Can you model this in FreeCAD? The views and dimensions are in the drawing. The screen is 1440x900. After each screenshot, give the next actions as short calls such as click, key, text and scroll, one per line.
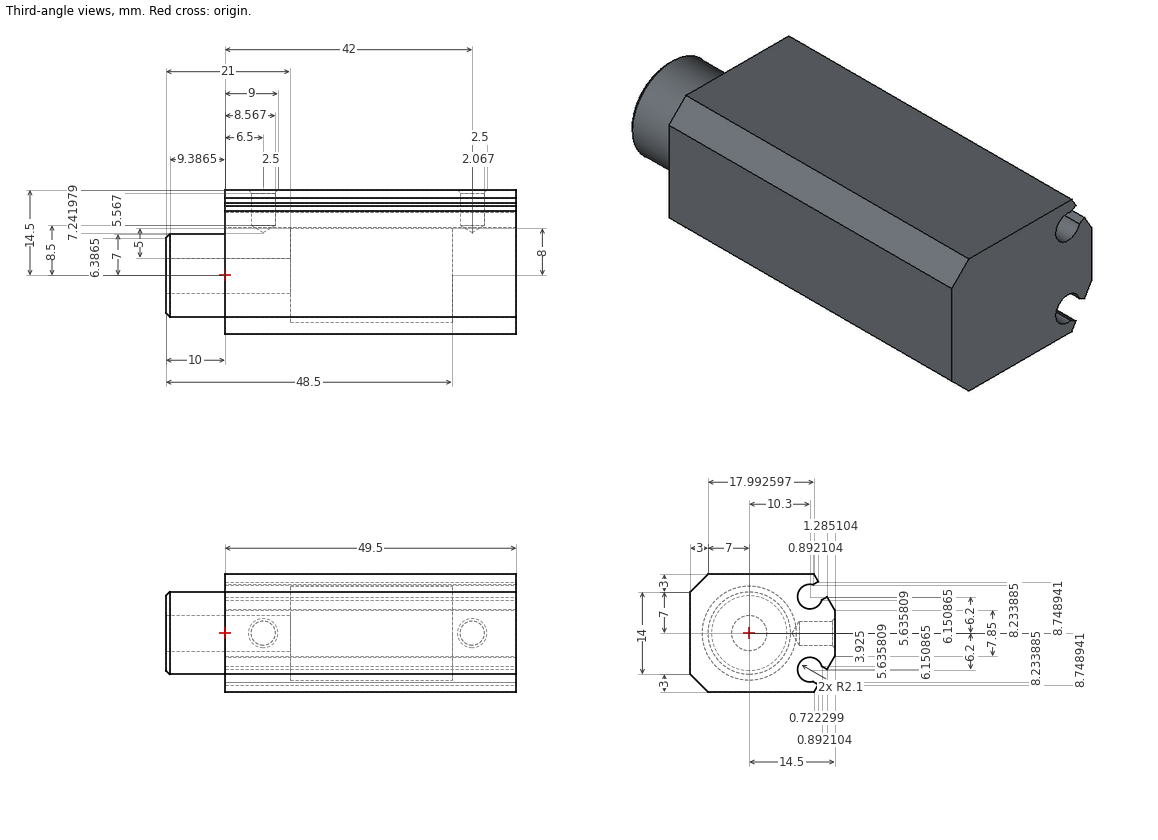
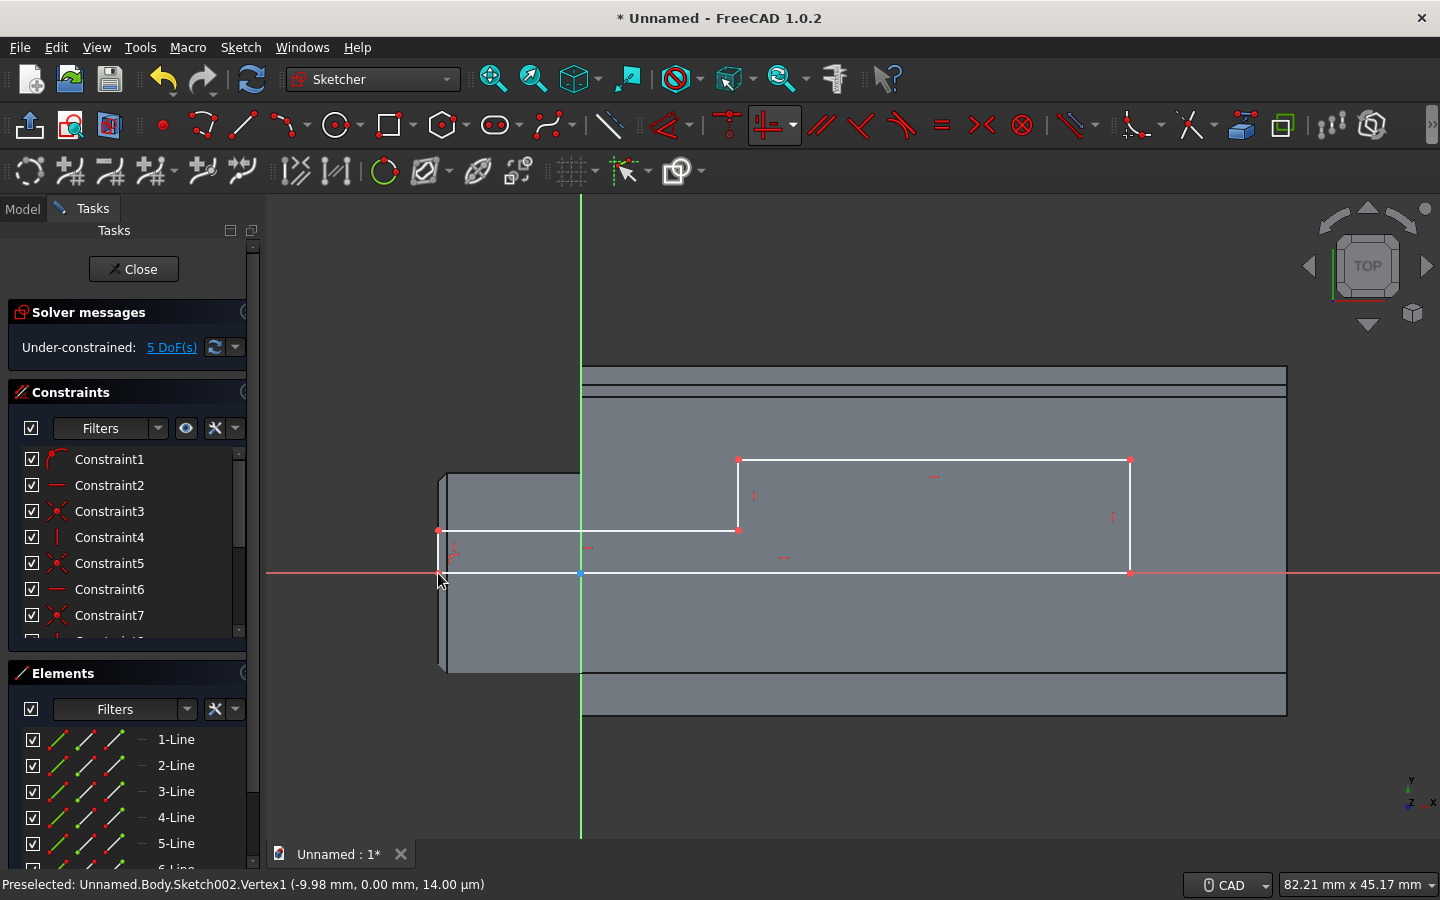
click(664, 126)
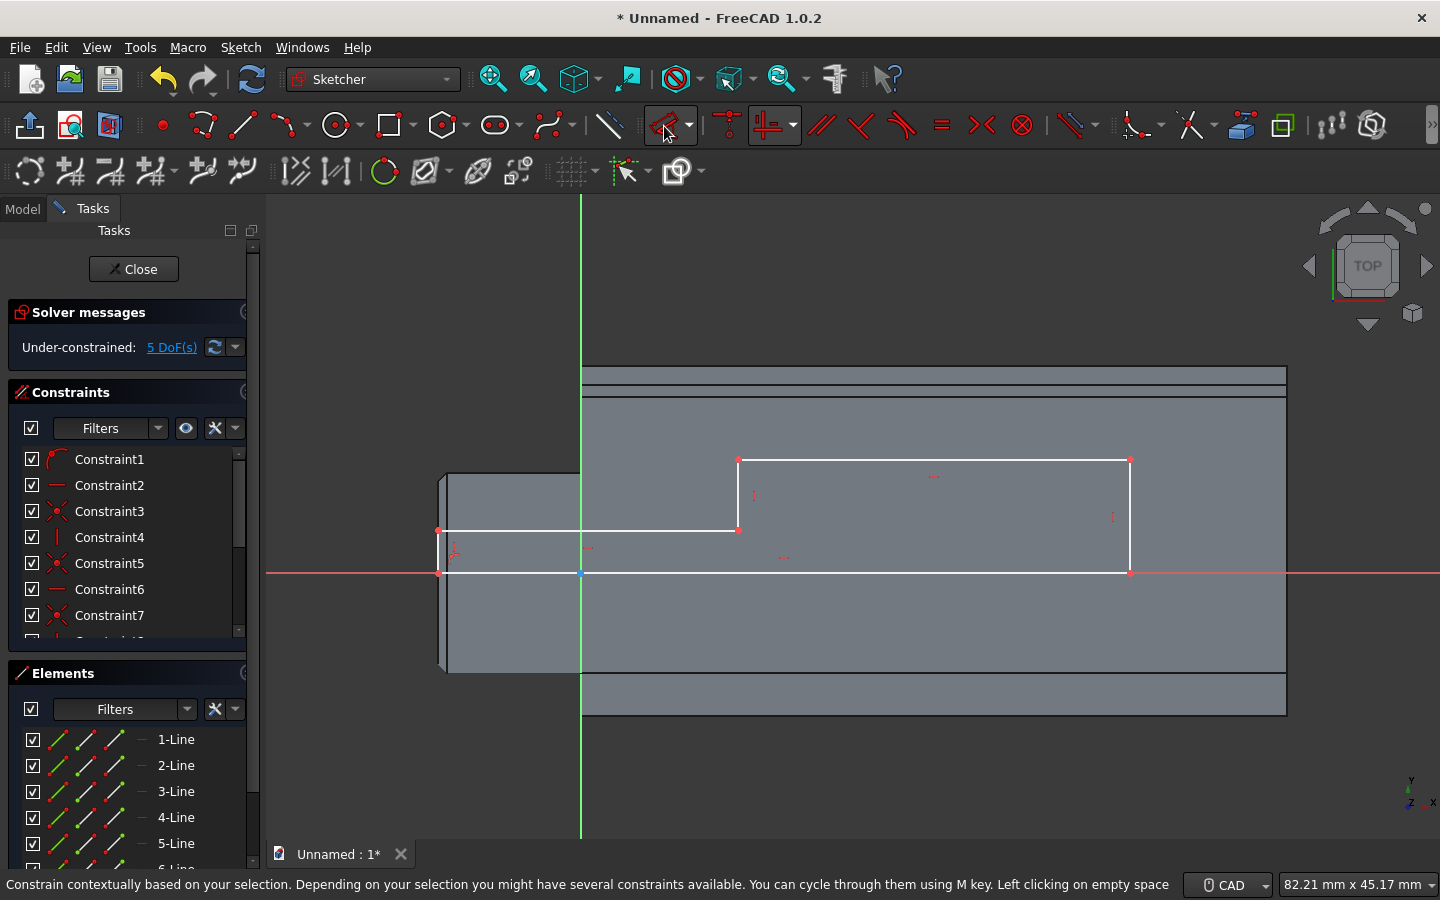
click(1130, 539)
click(1164, 517)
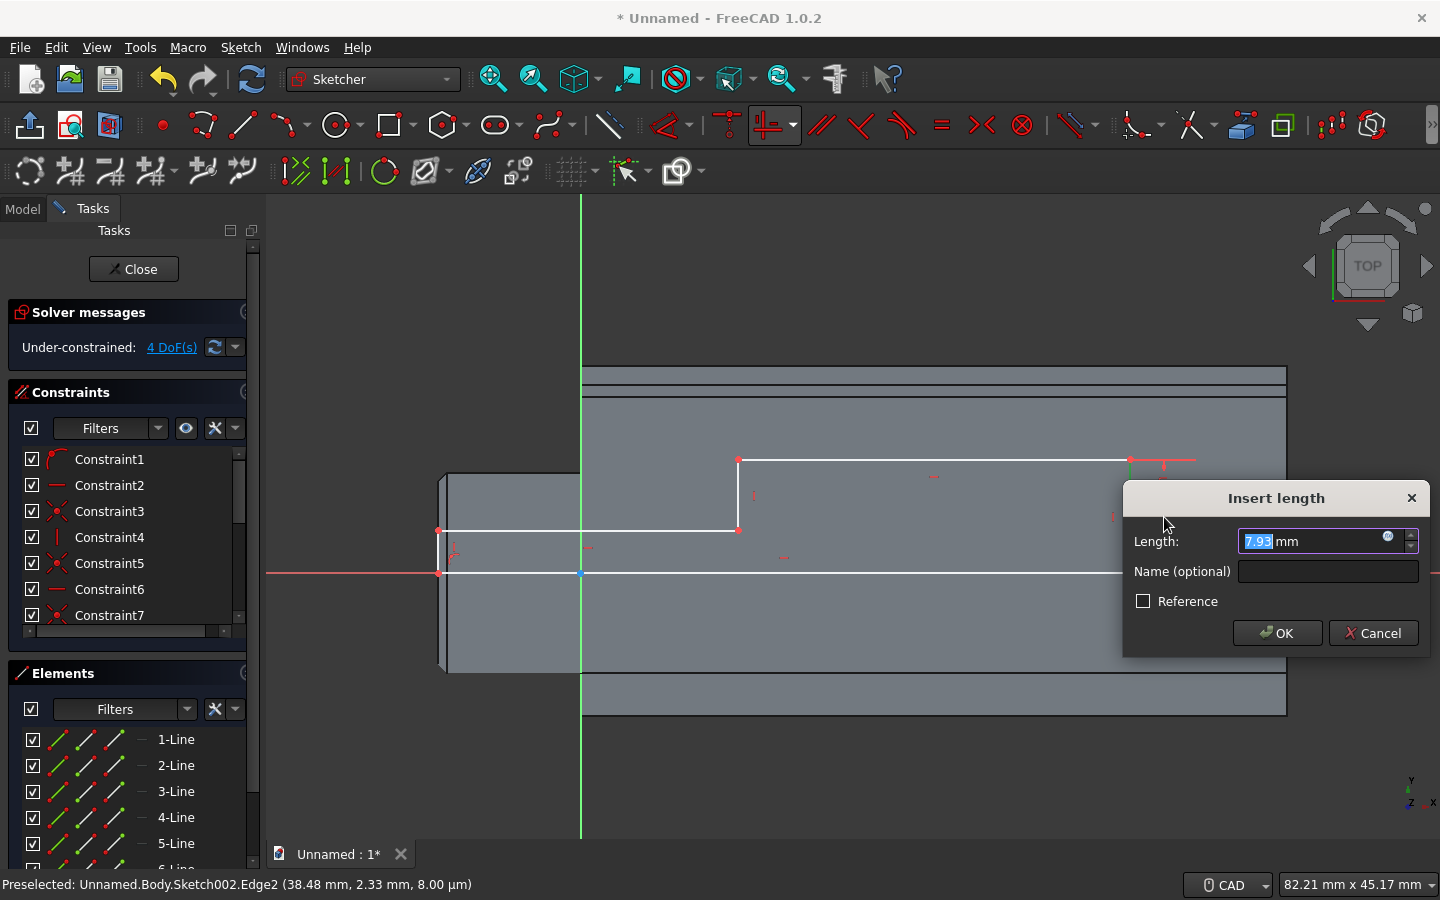
text(8)
key(Return)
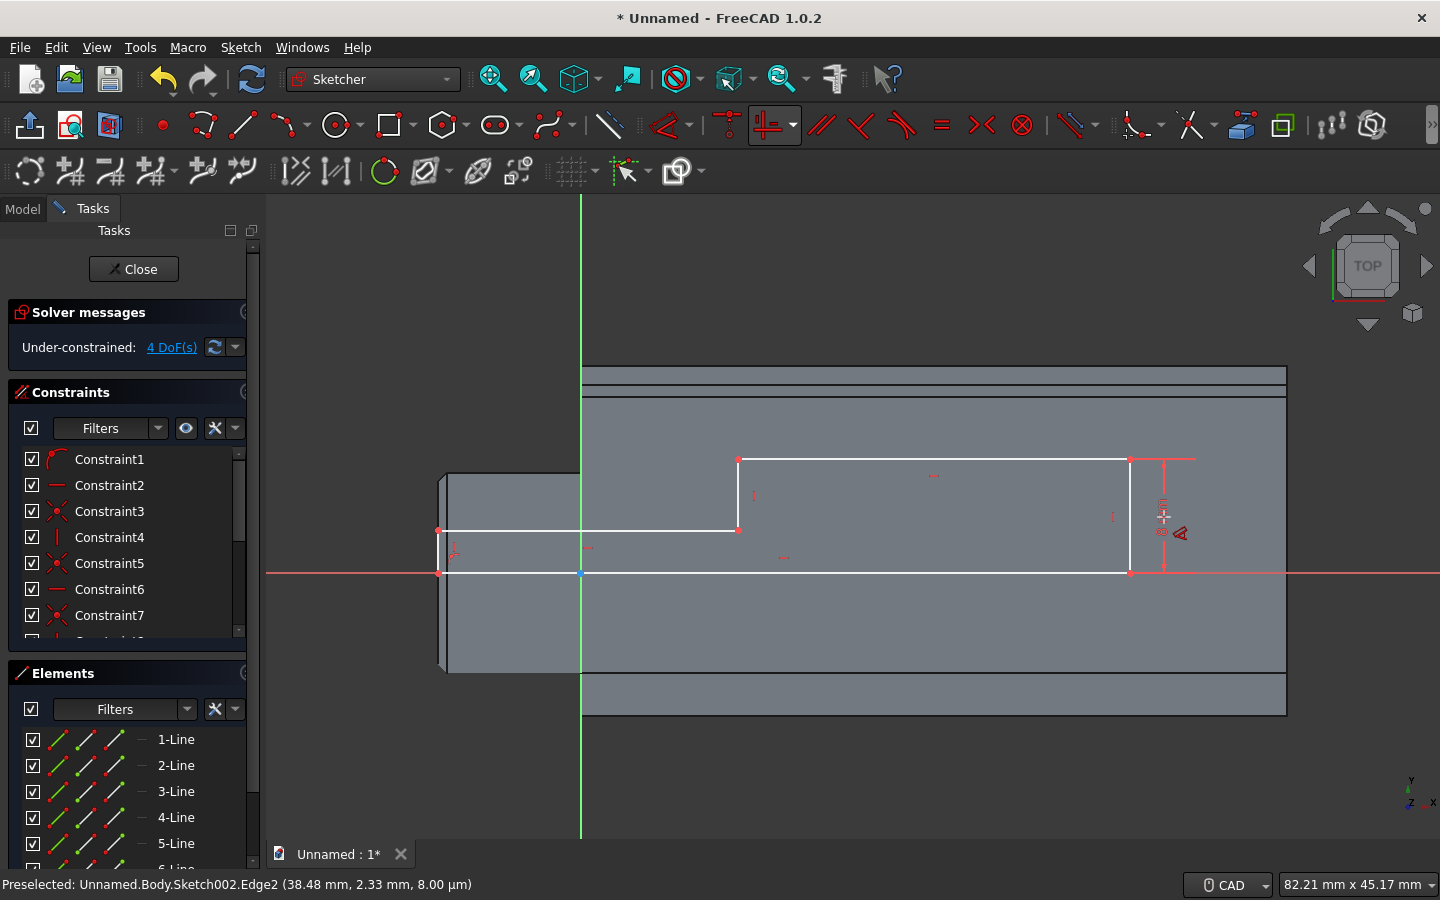
click(738, 481)
click(704, 495)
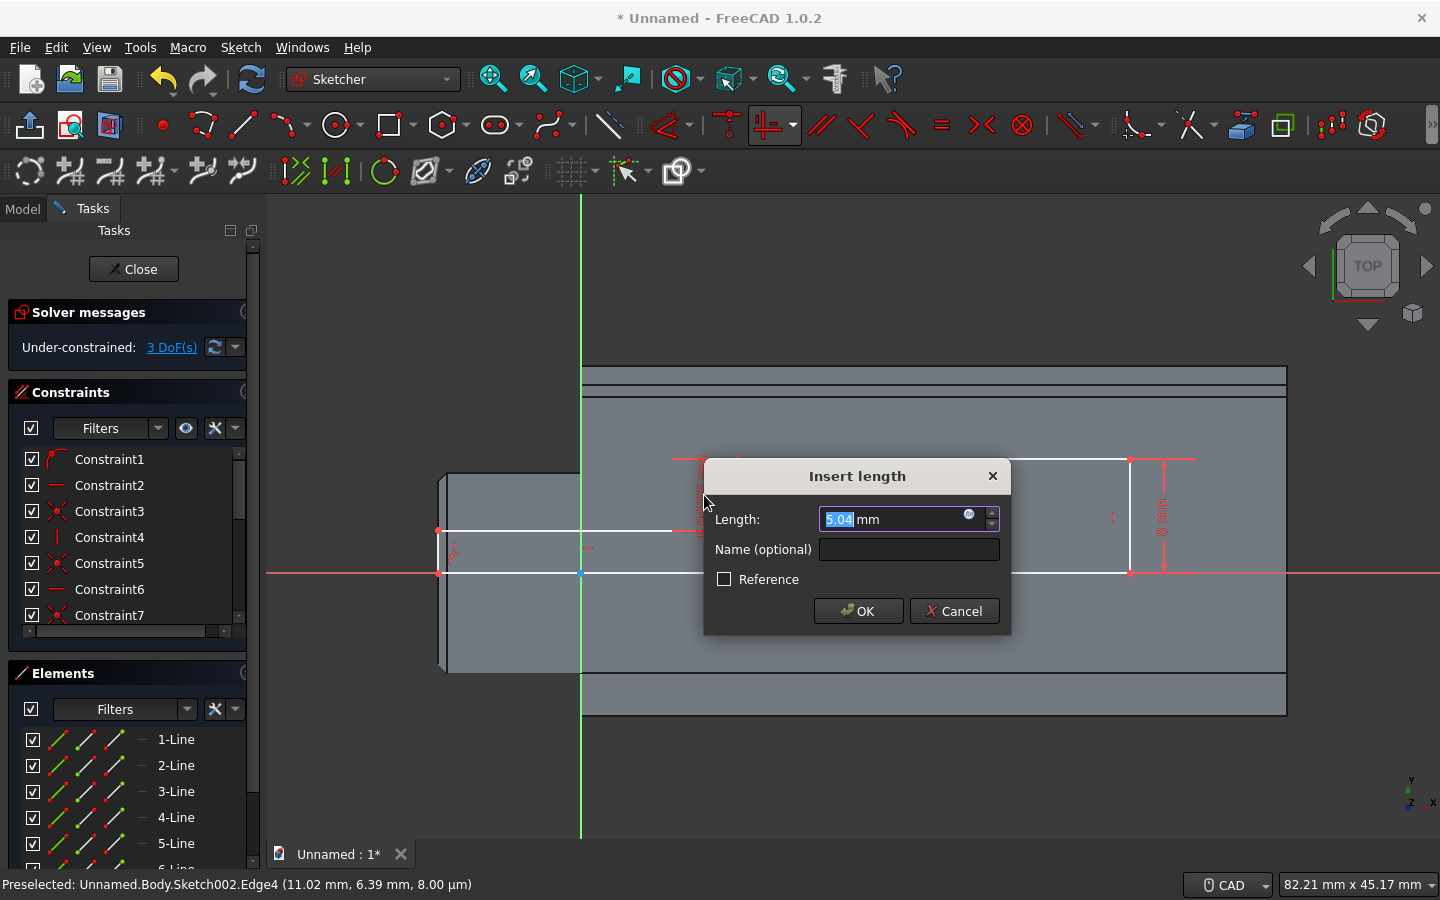
text(5)
key(Return)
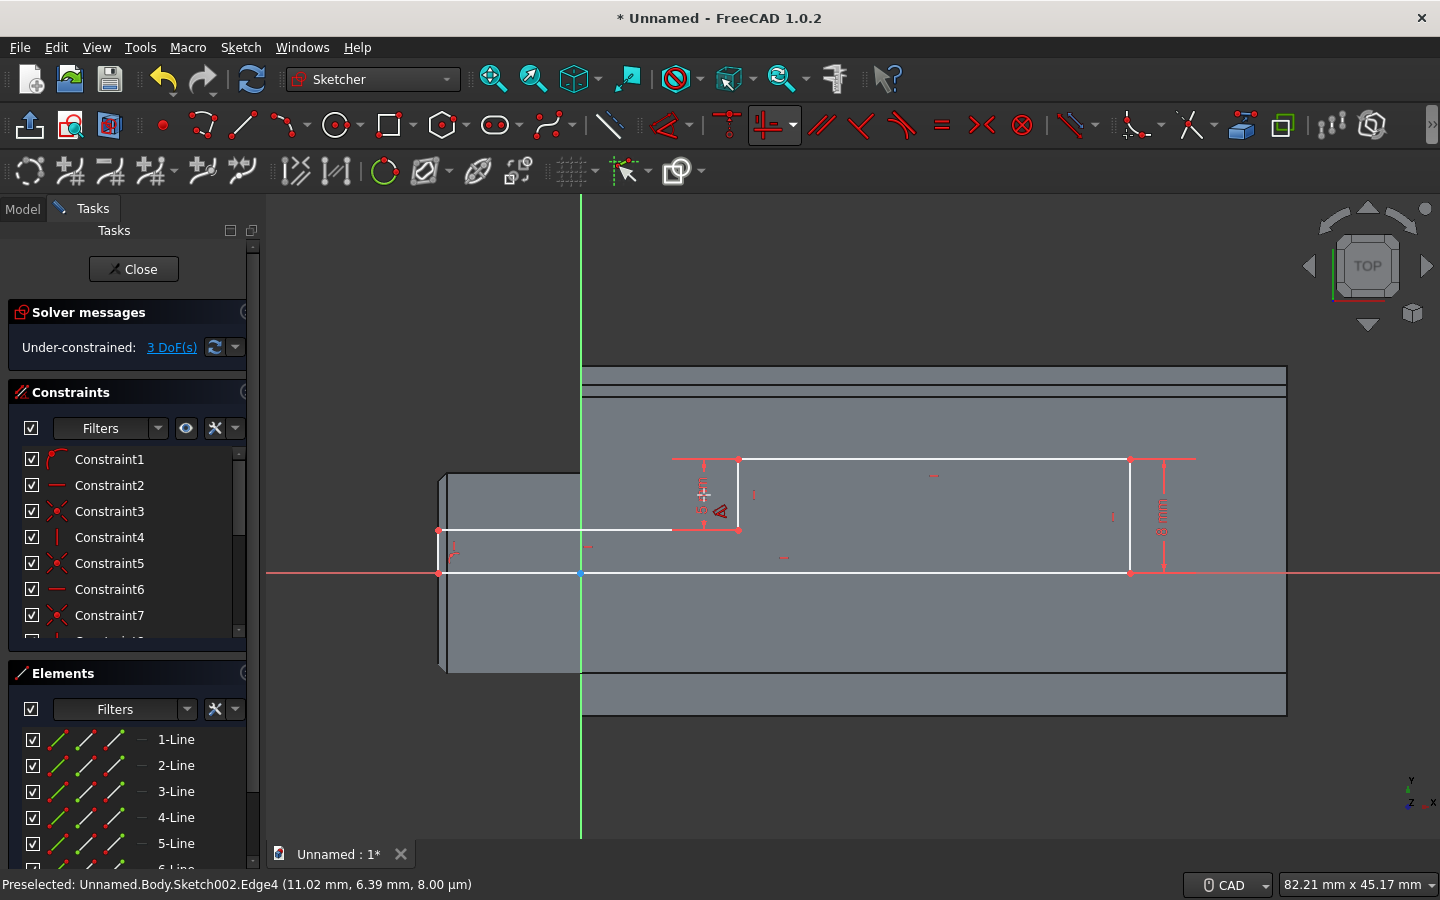
click(648, 530)
click(519, 496)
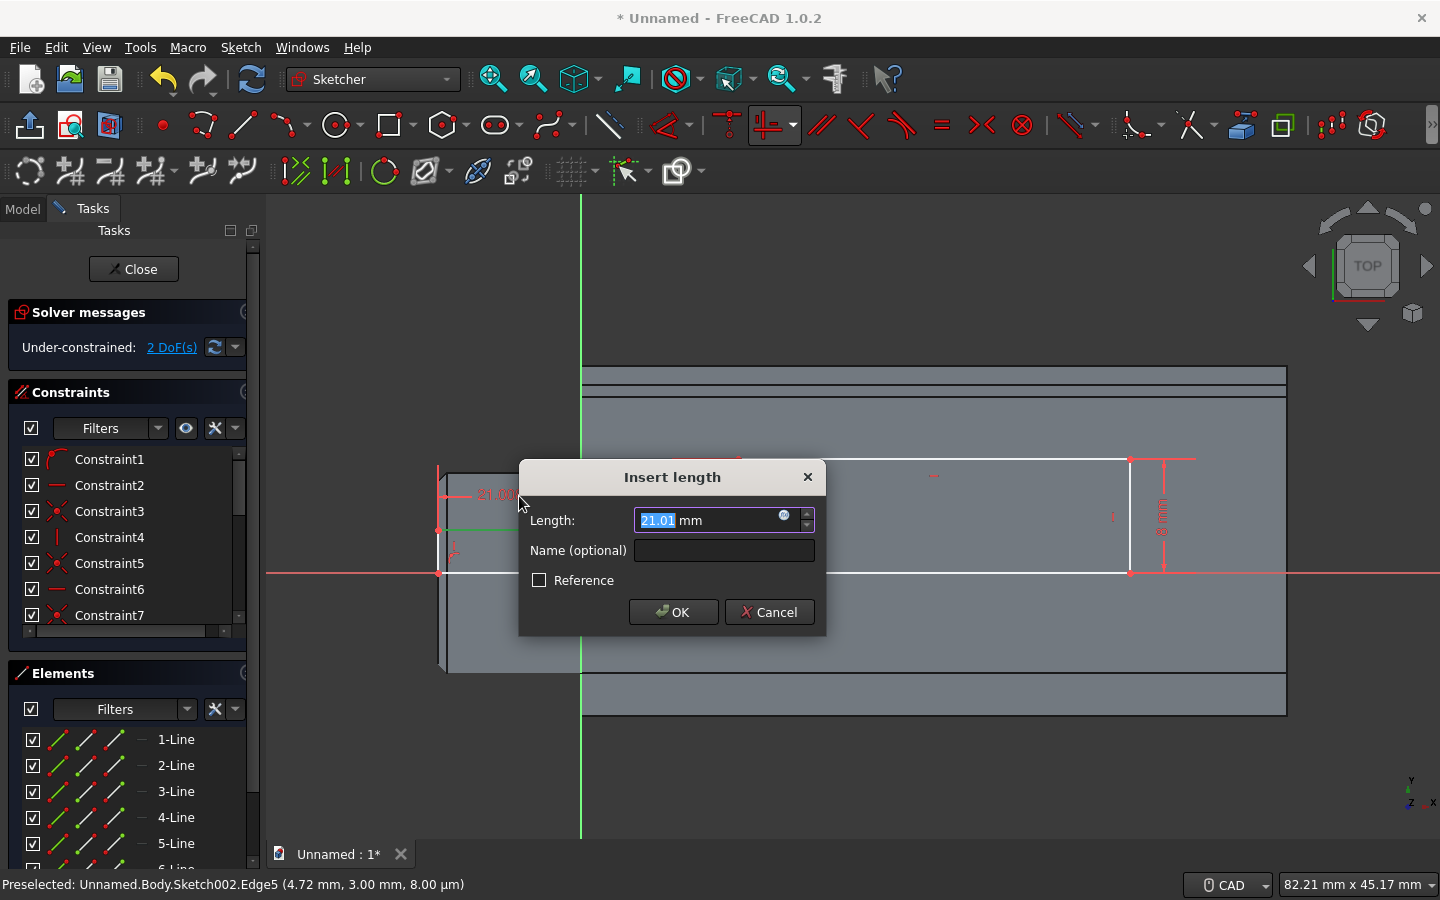
text(21)
key(Return)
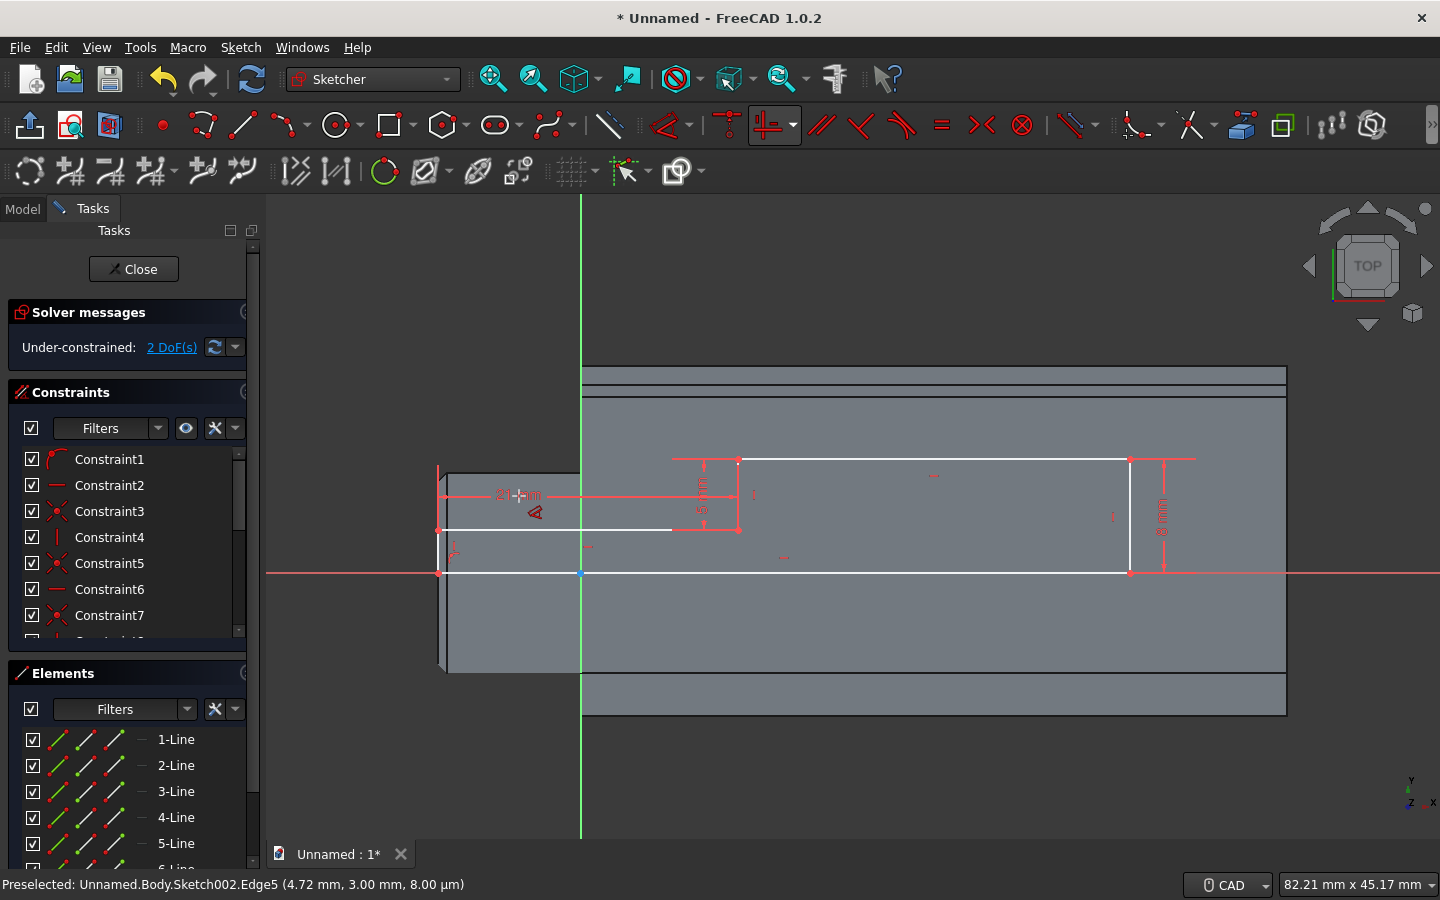
click(438, 573)
click(509, 607)